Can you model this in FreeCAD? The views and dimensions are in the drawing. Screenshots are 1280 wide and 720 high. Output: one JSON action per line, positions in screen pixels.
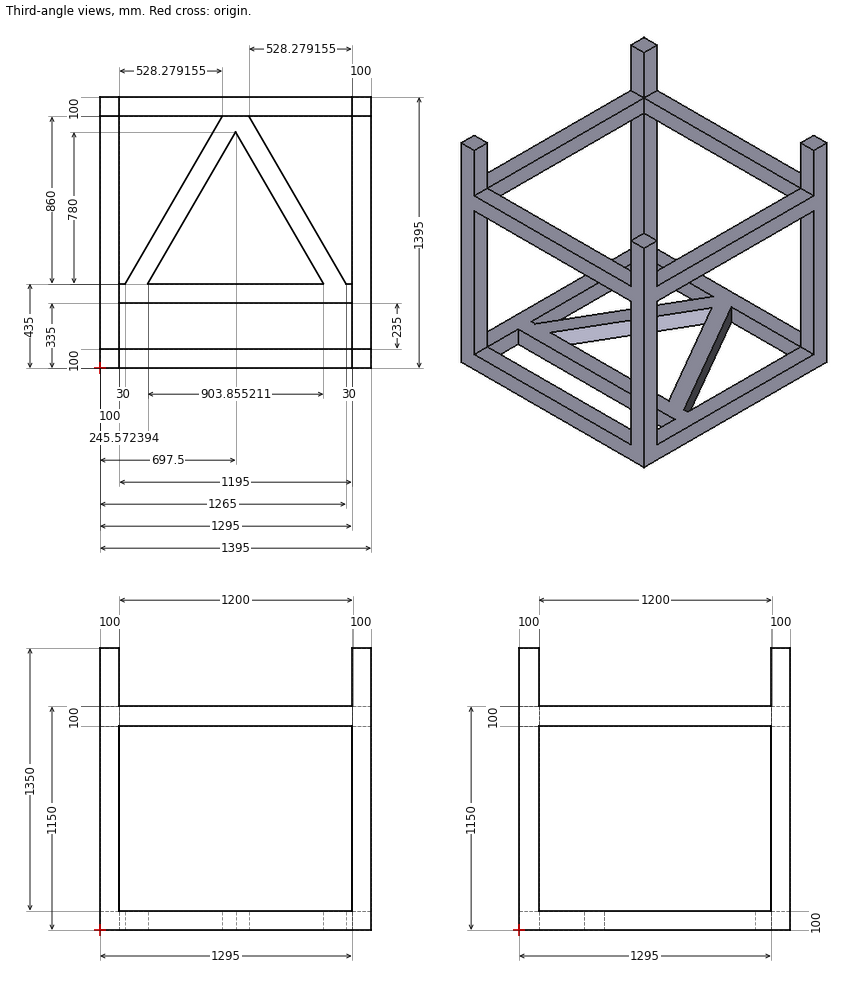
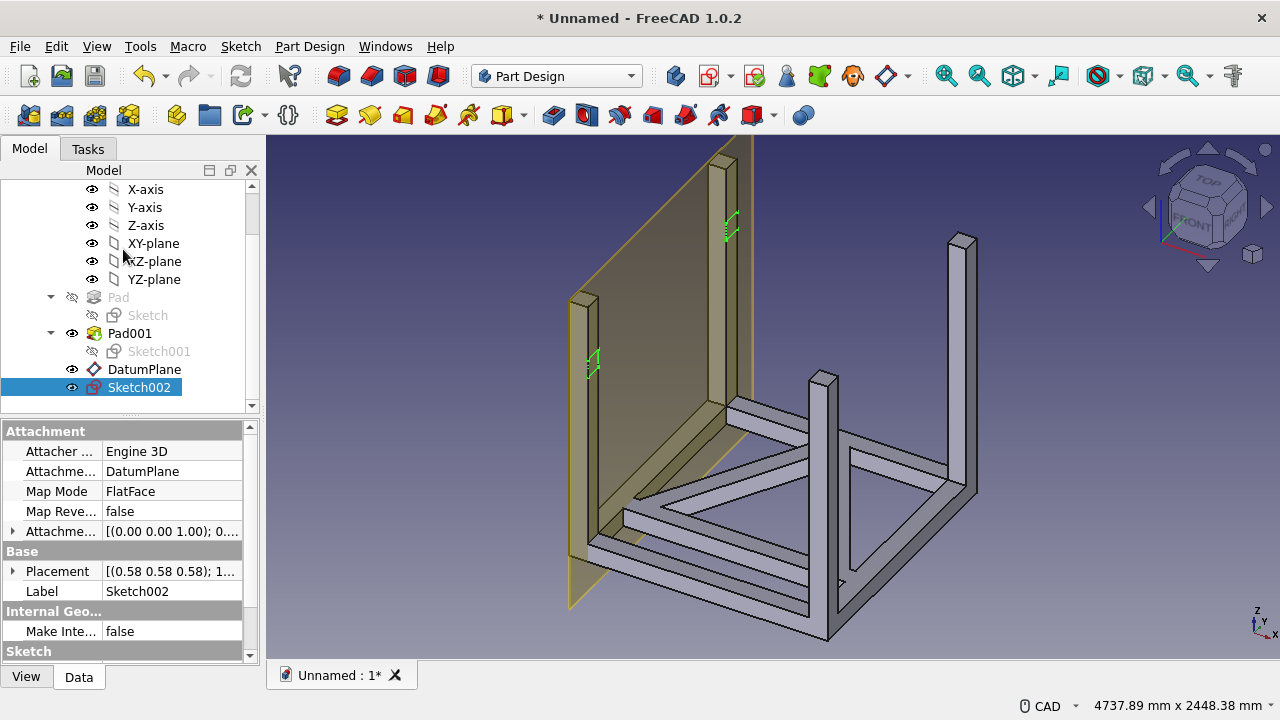
{"action": "left_click", "coordinate": [337, 116]}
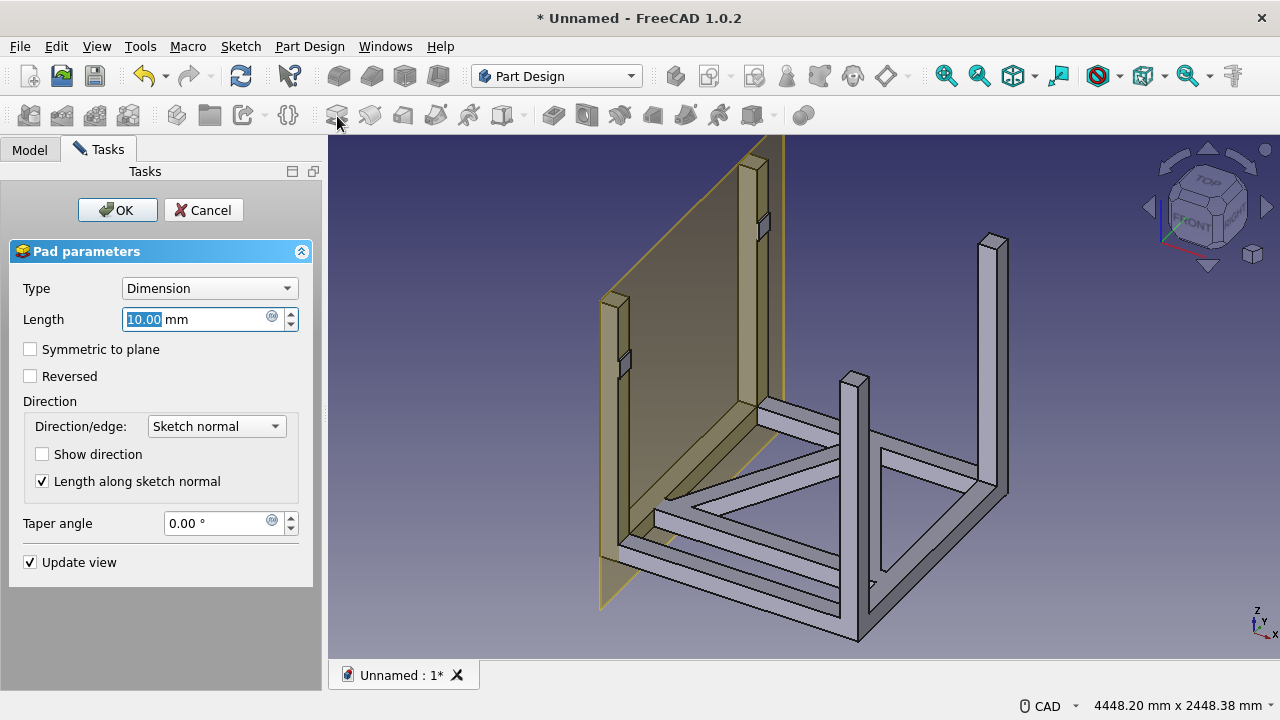
{"action": "type", "text": "1200"}
{"action": "key", "text": "Tab"}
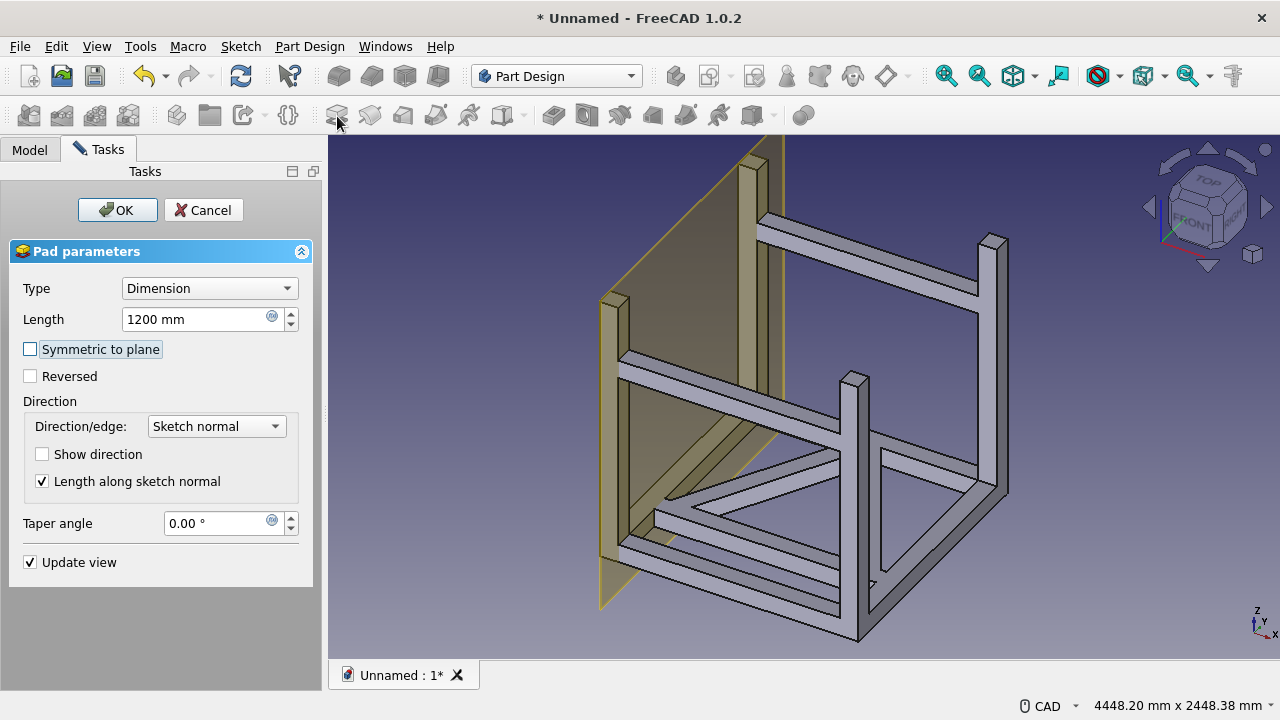
{"action": "left_click", "coordinate": [118, 210]}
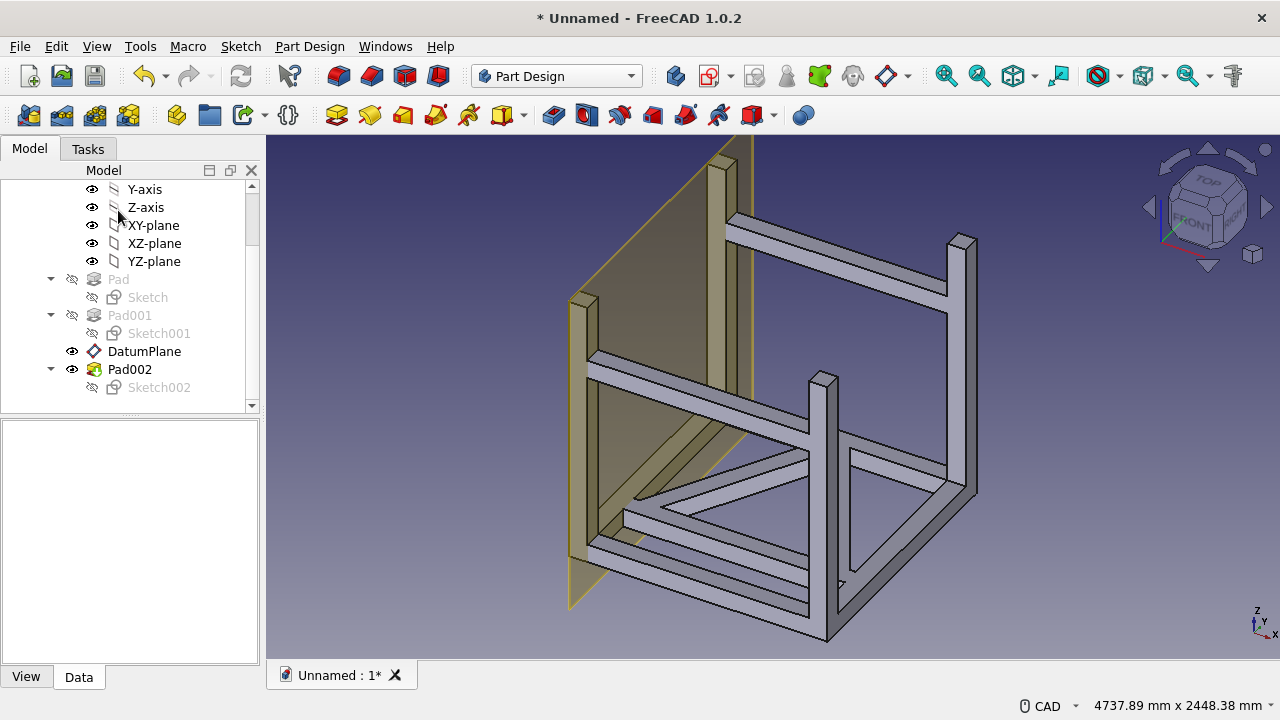
{"action": "left_click", "coordinate": [117, 351]}
{"action": "key", "text": "space"}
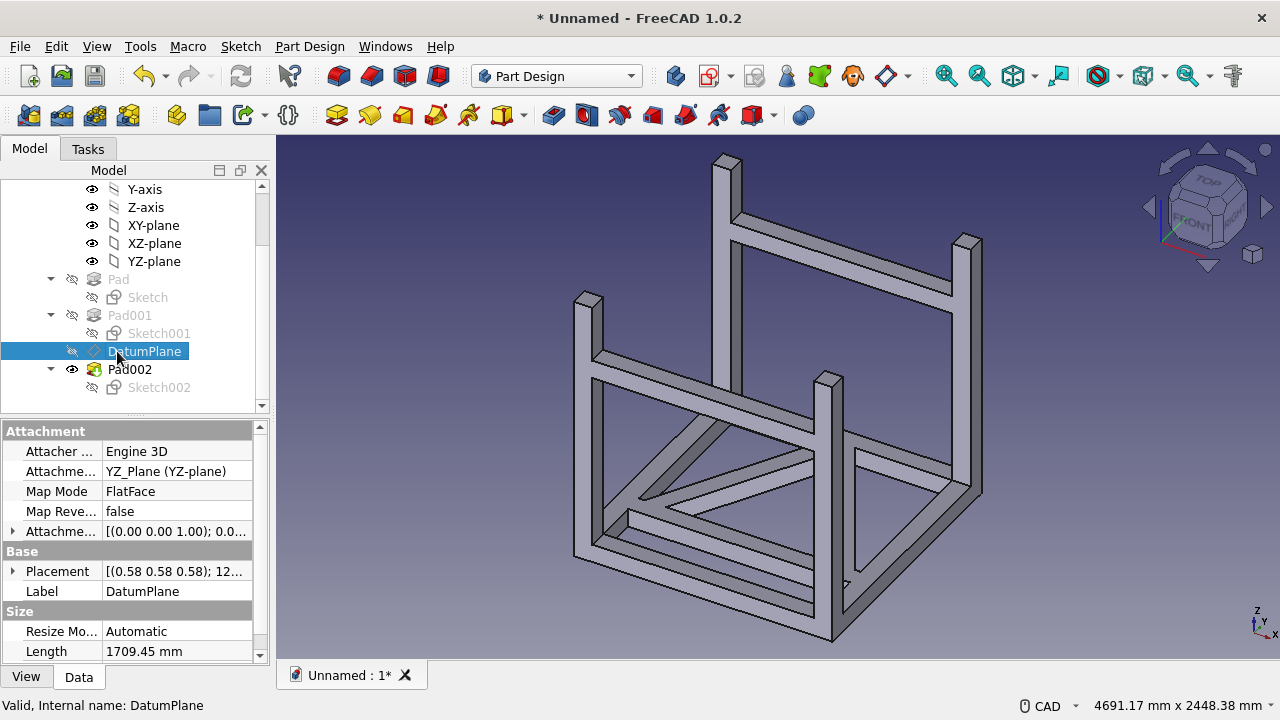
{"action": "scroll", "coordinate": [161, 293], "scroll_direction": "down", "scroll_amount": 3}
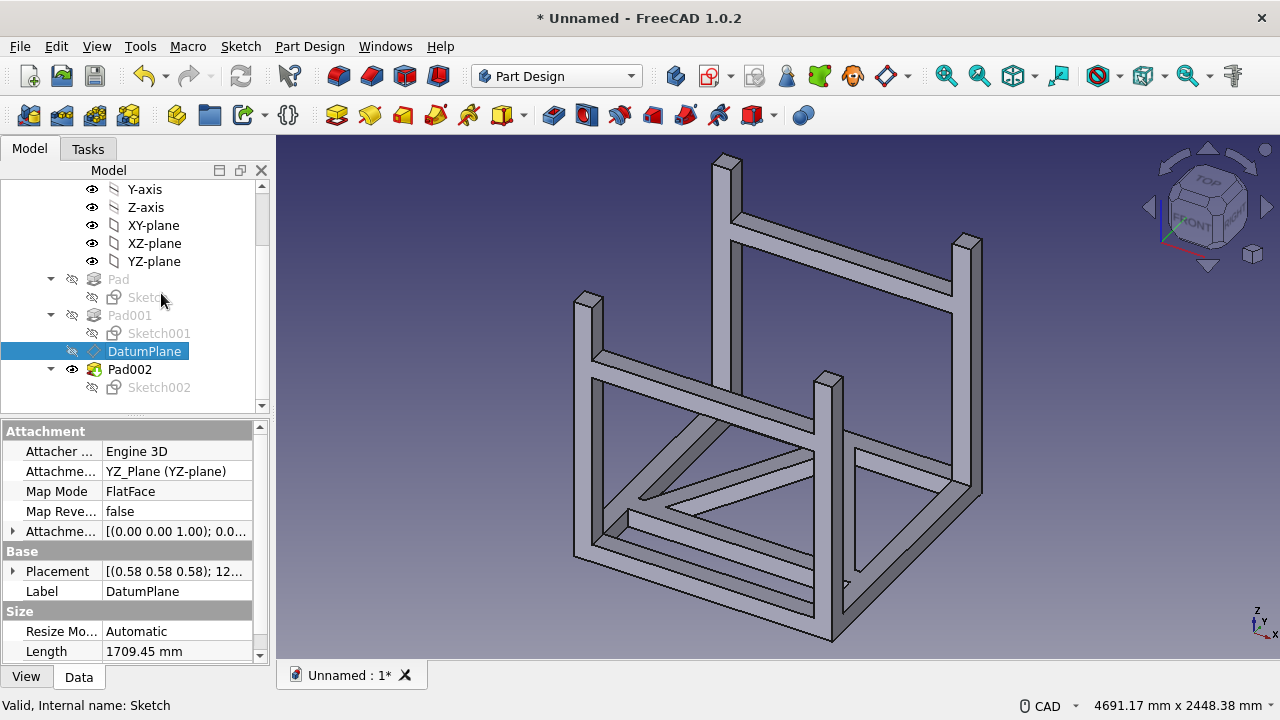
{"action": "scroll", "coordinate": [161, 293], "scroll_direction": "up", "scroll_amount": 15}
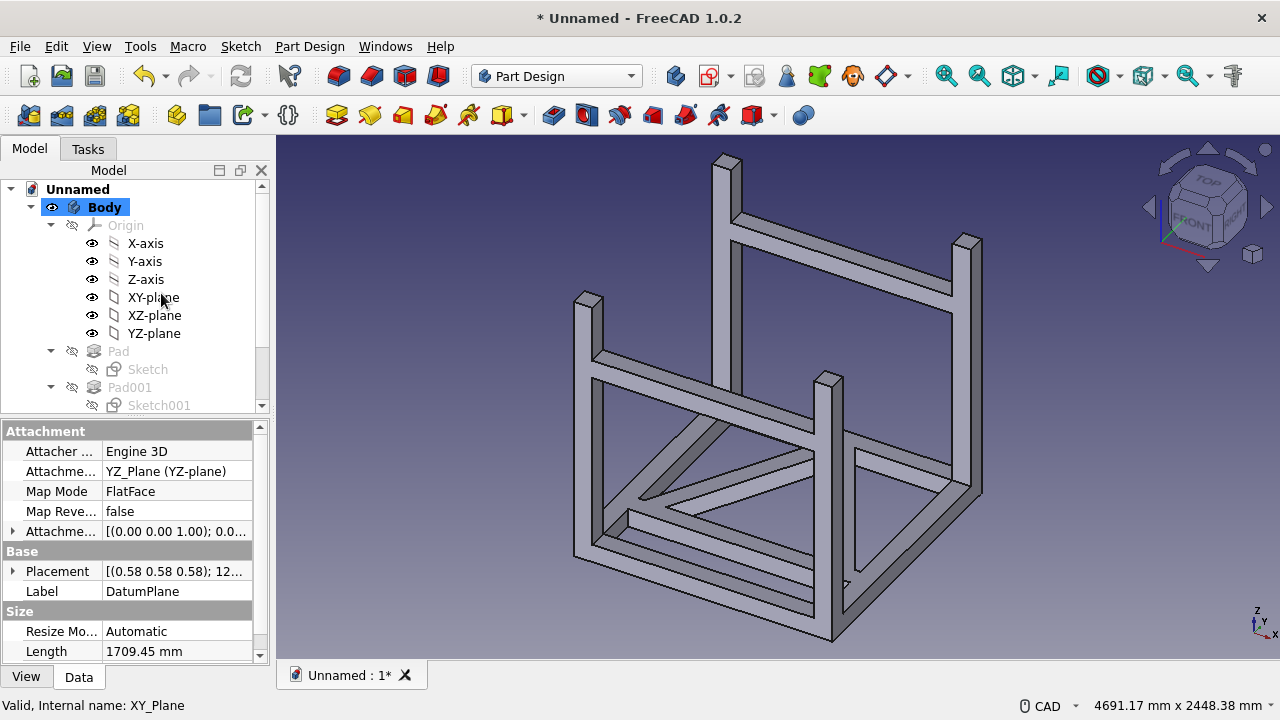
{"action": "left_click", "coordinate": [137, 315]}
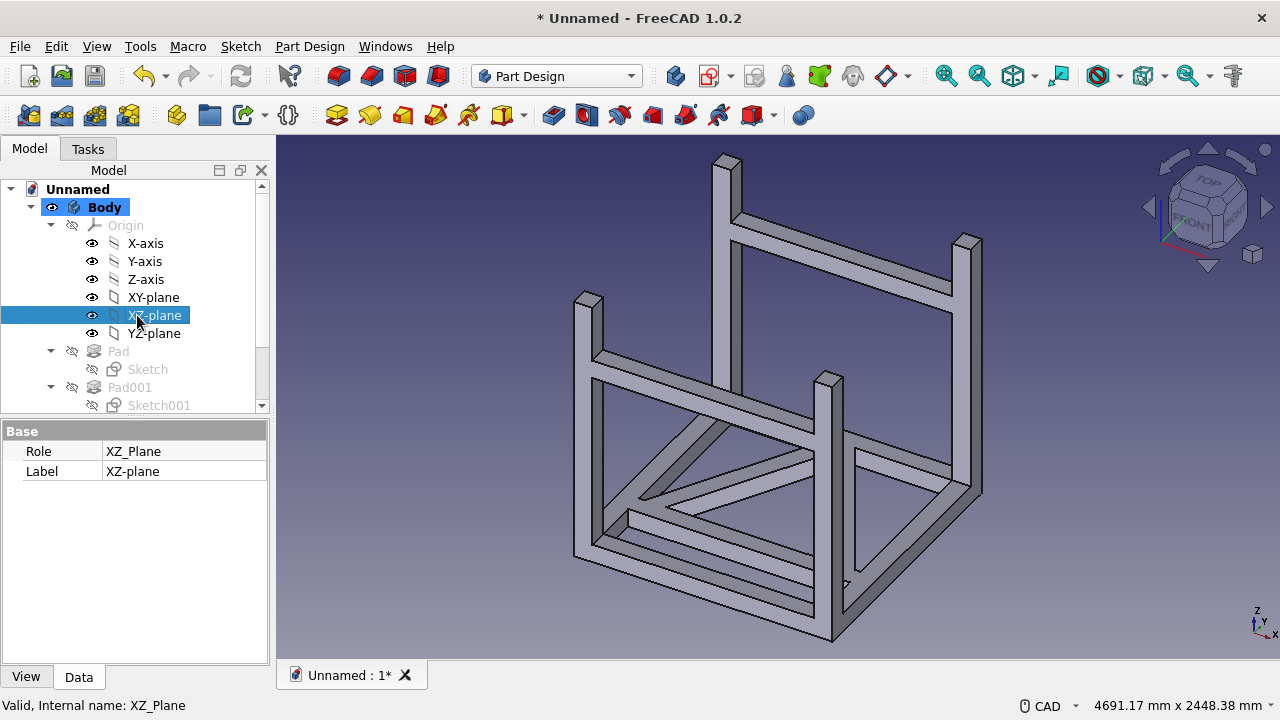
{"action": "left_click", "coordinate": [886, 76]}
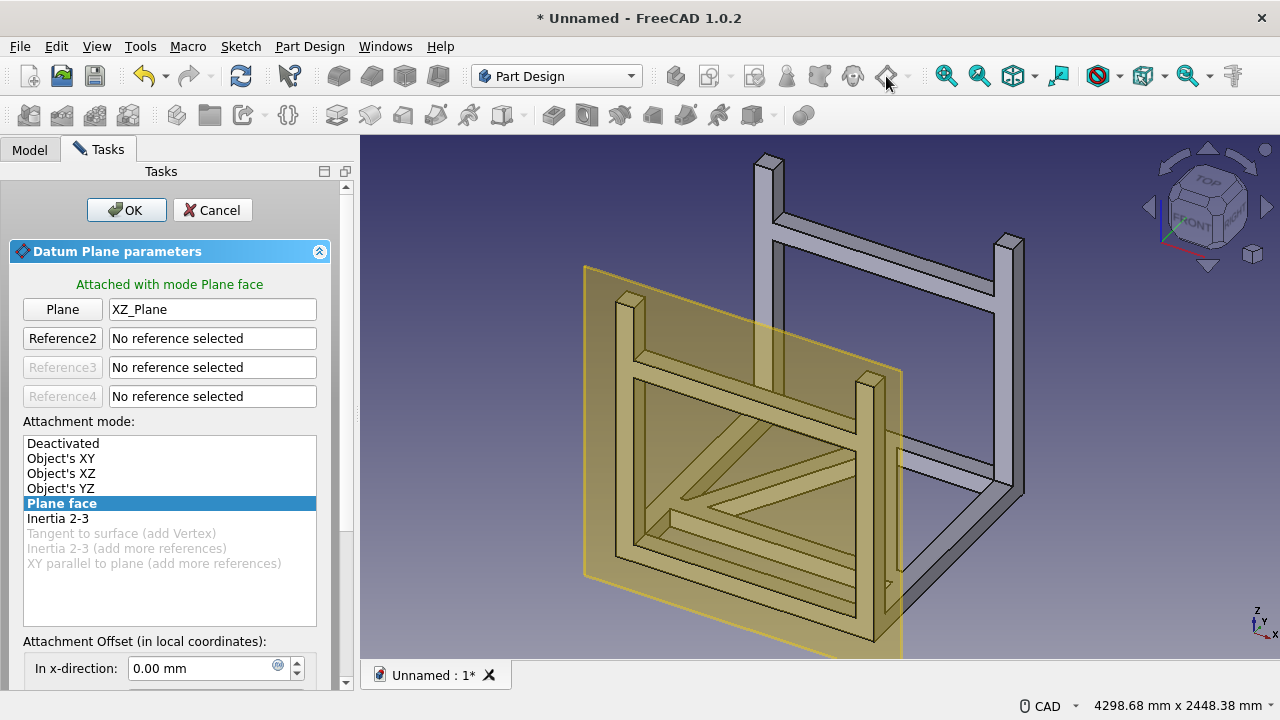
{"action": "scroll", "coordinate": [346, 436], "scroll_direction": "down", "scroll_amount": 2}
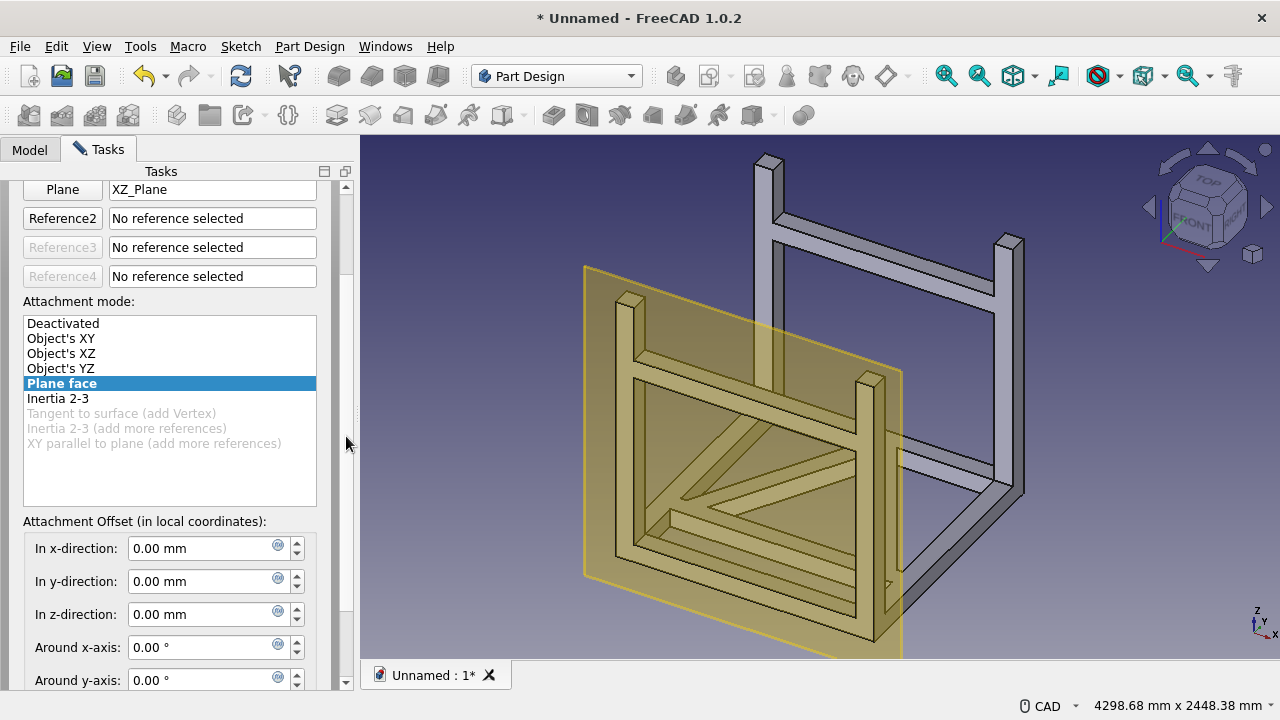
{"action": "triple_click", "coordinate": [210, 614]}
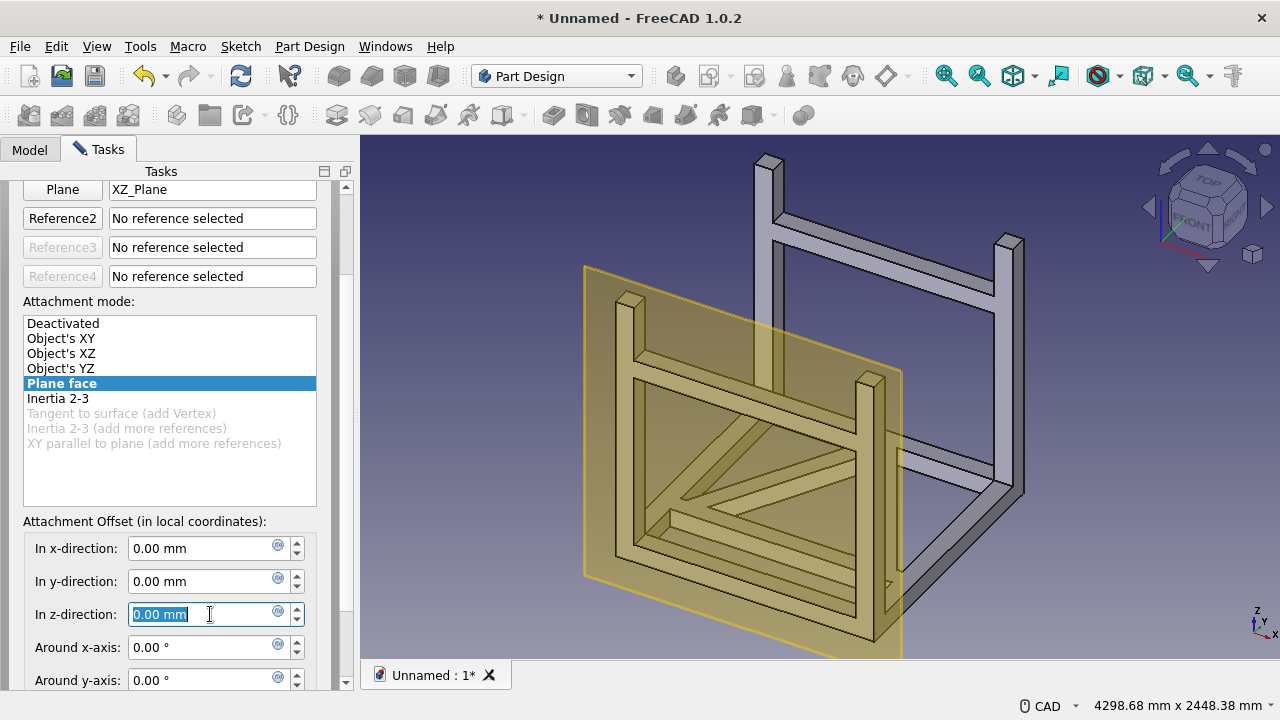
{"action": "type", "text": "-100"}
{"action": "key", "text": "Tab"}